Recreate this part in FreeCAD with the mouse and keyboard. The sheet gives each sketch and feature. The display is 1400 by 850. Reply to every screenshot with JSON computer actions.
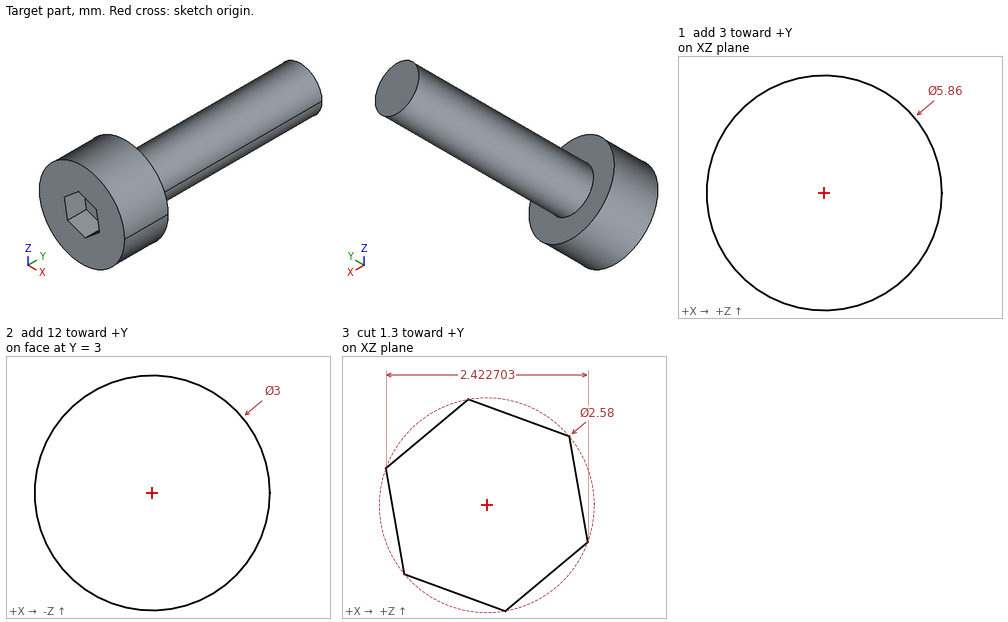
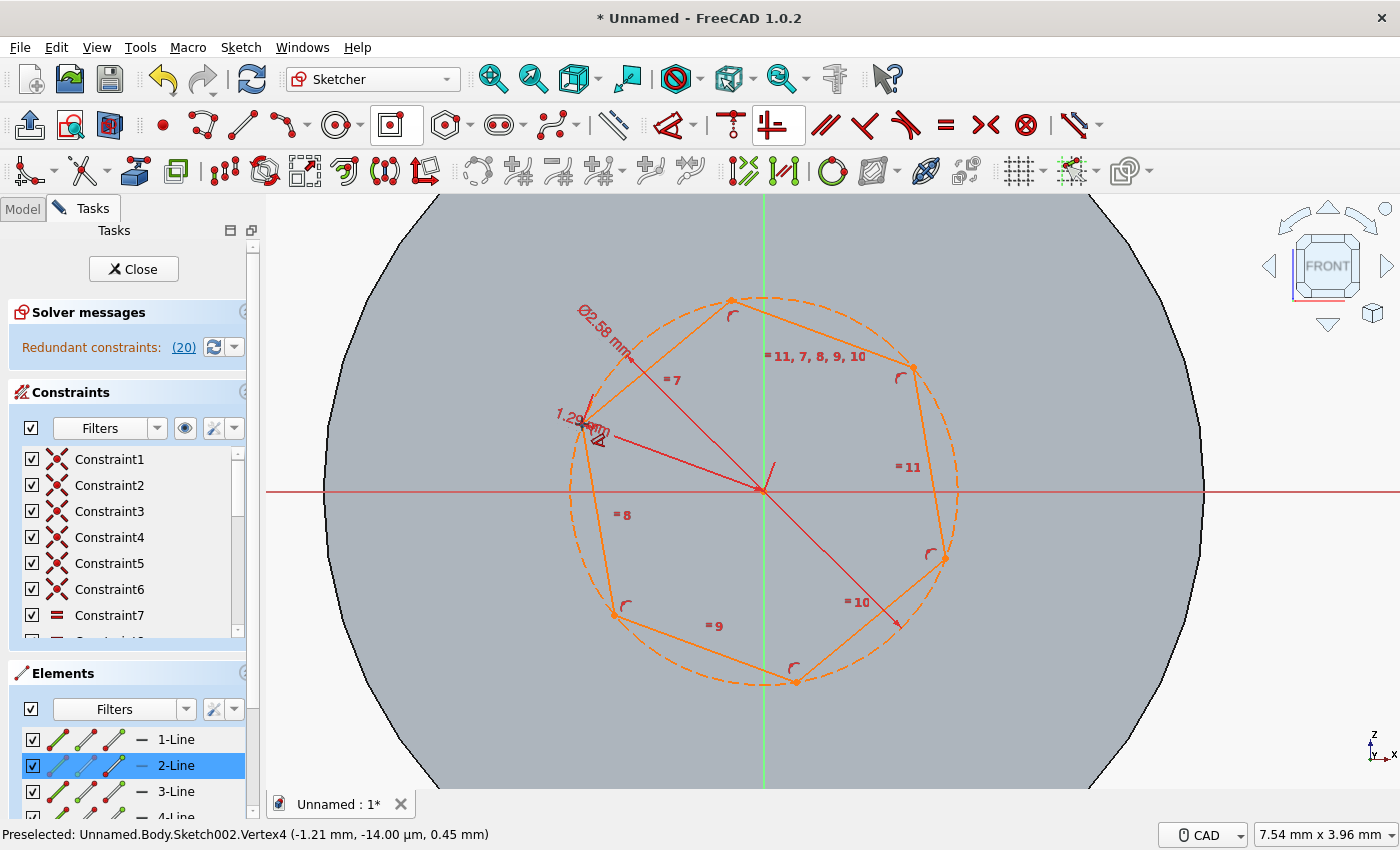
{"action": "left_click", "coordinate": [946, 559]}
{"action": "left_click", "coordinate": [680, 593]}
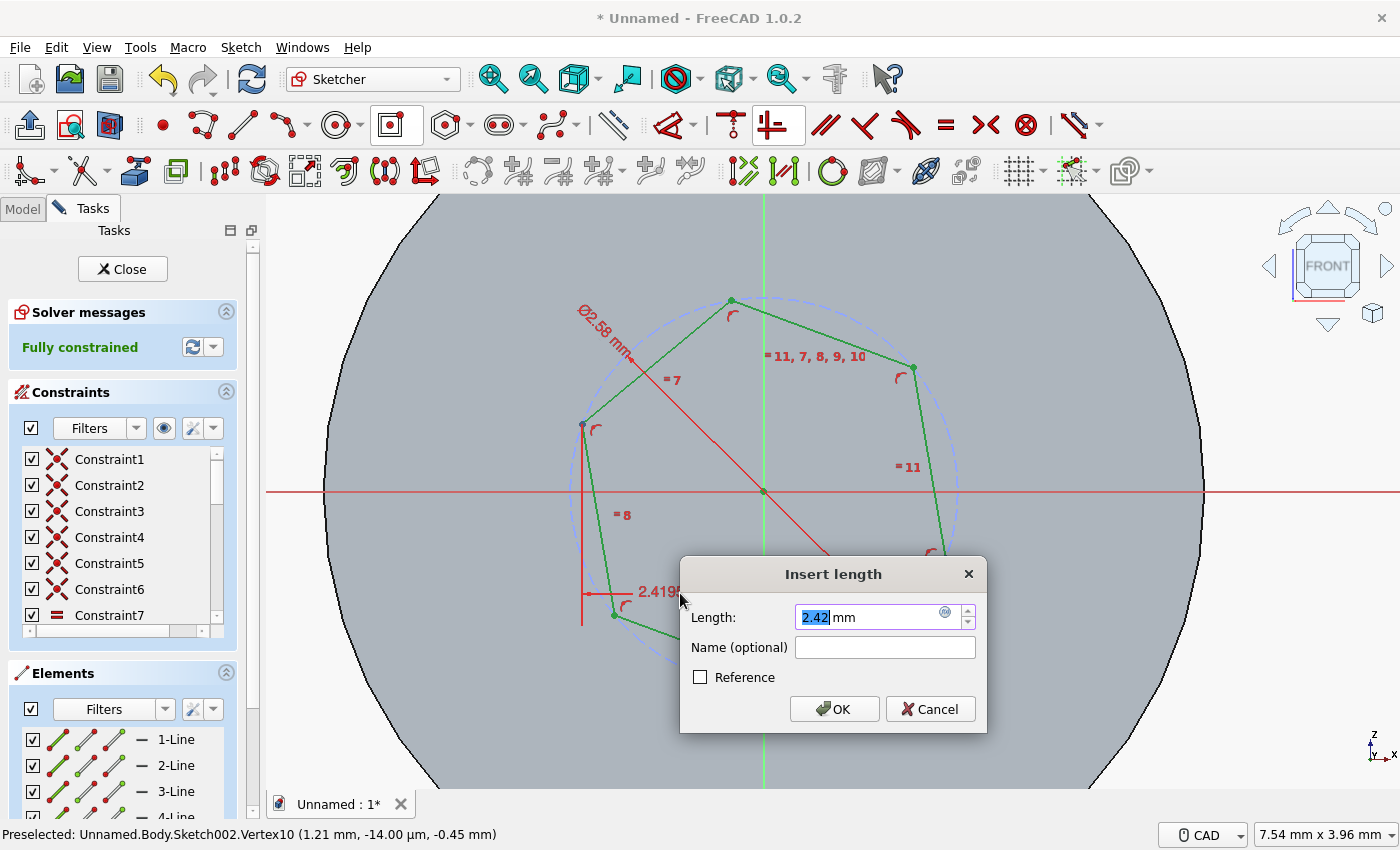
{"action": "type", "text": "2.422703"}
{"action": "key", "text": "Return"}
{"action": "key", "text": "Escape"}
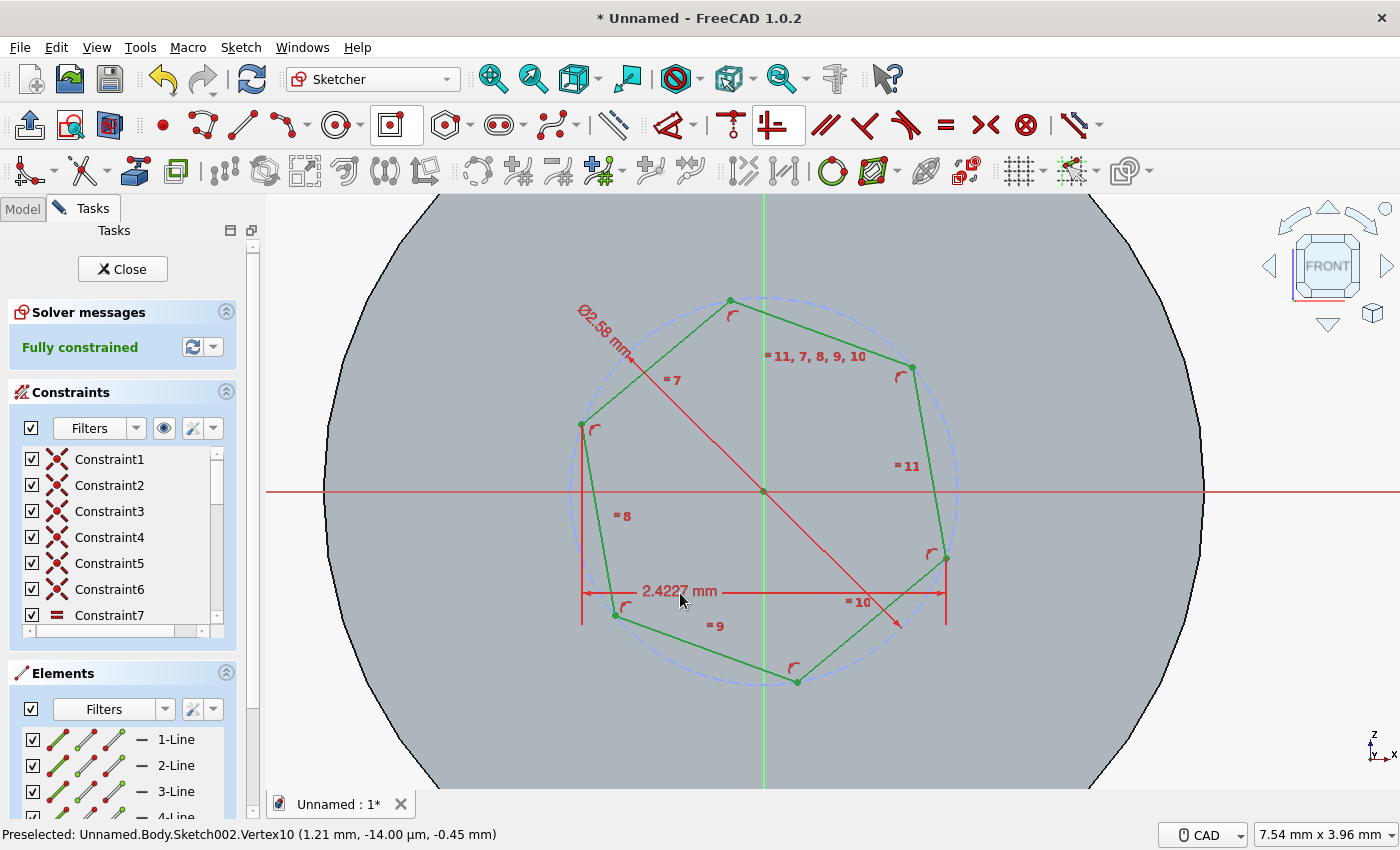
{"action": "left_click", "coordinate": [123, 269]}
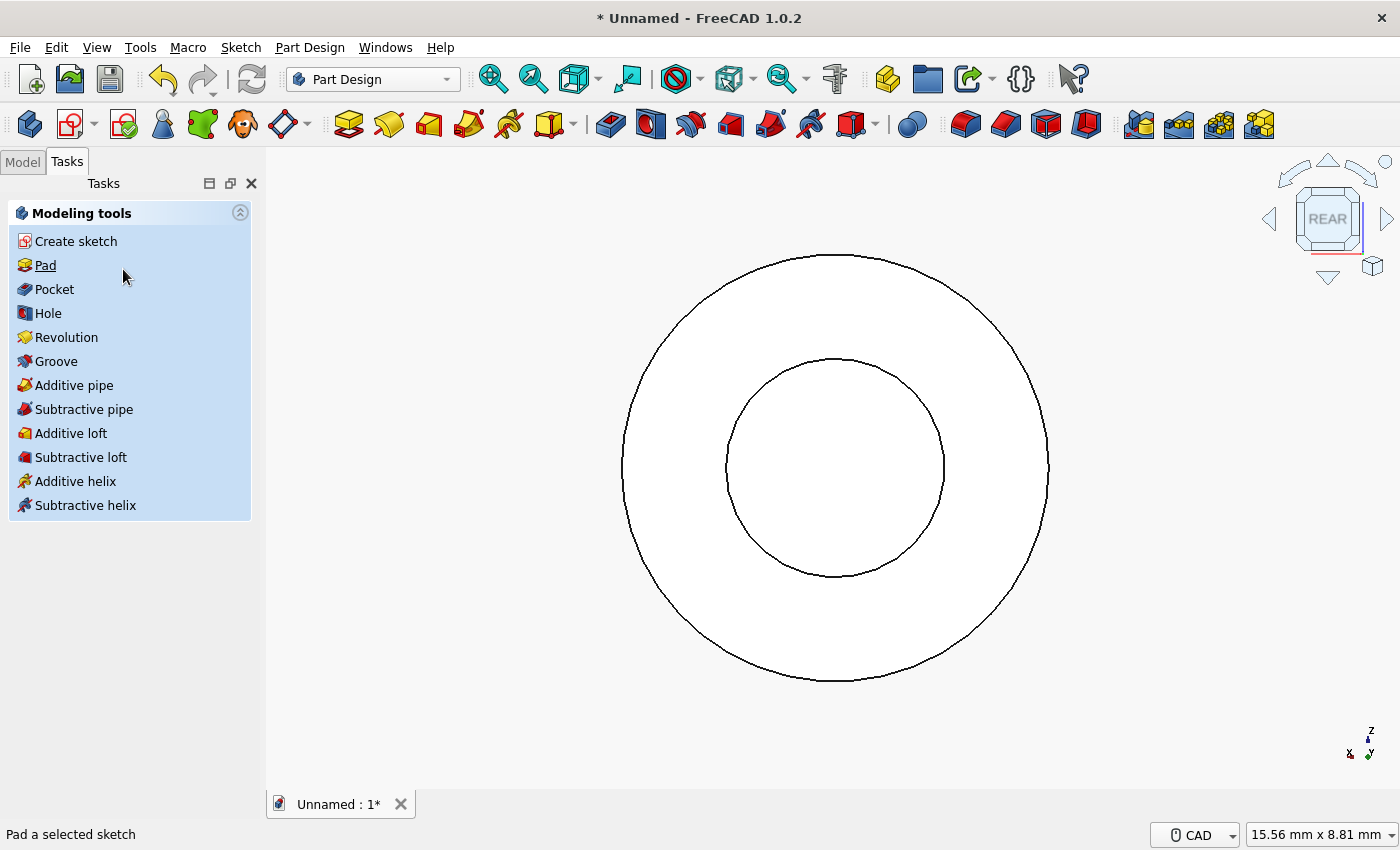
{"action": "left_click", "coordinate": [612, 124]}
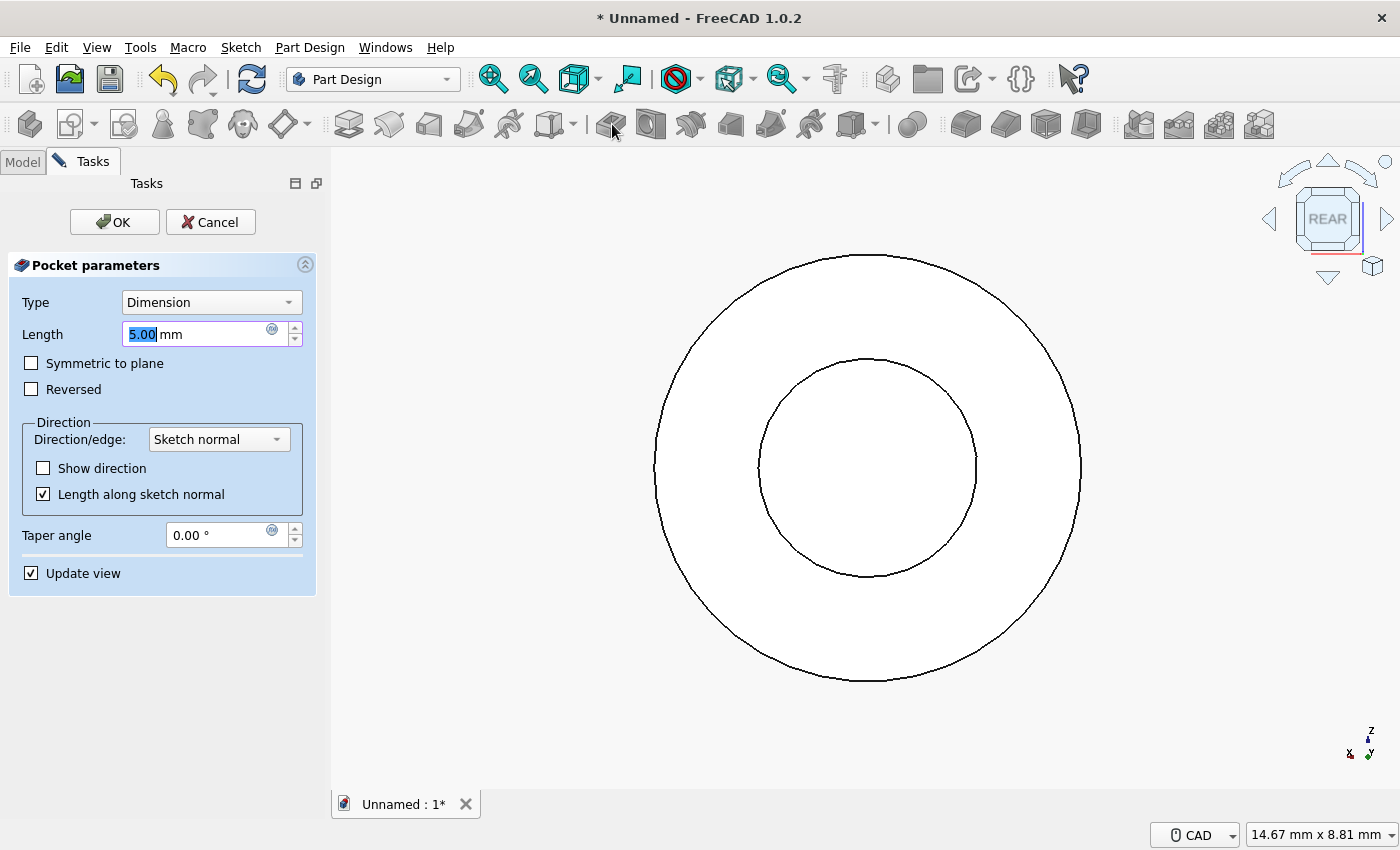
{"action": "type", "text": "1.3"}
{"action": "key", "text": "Tab"}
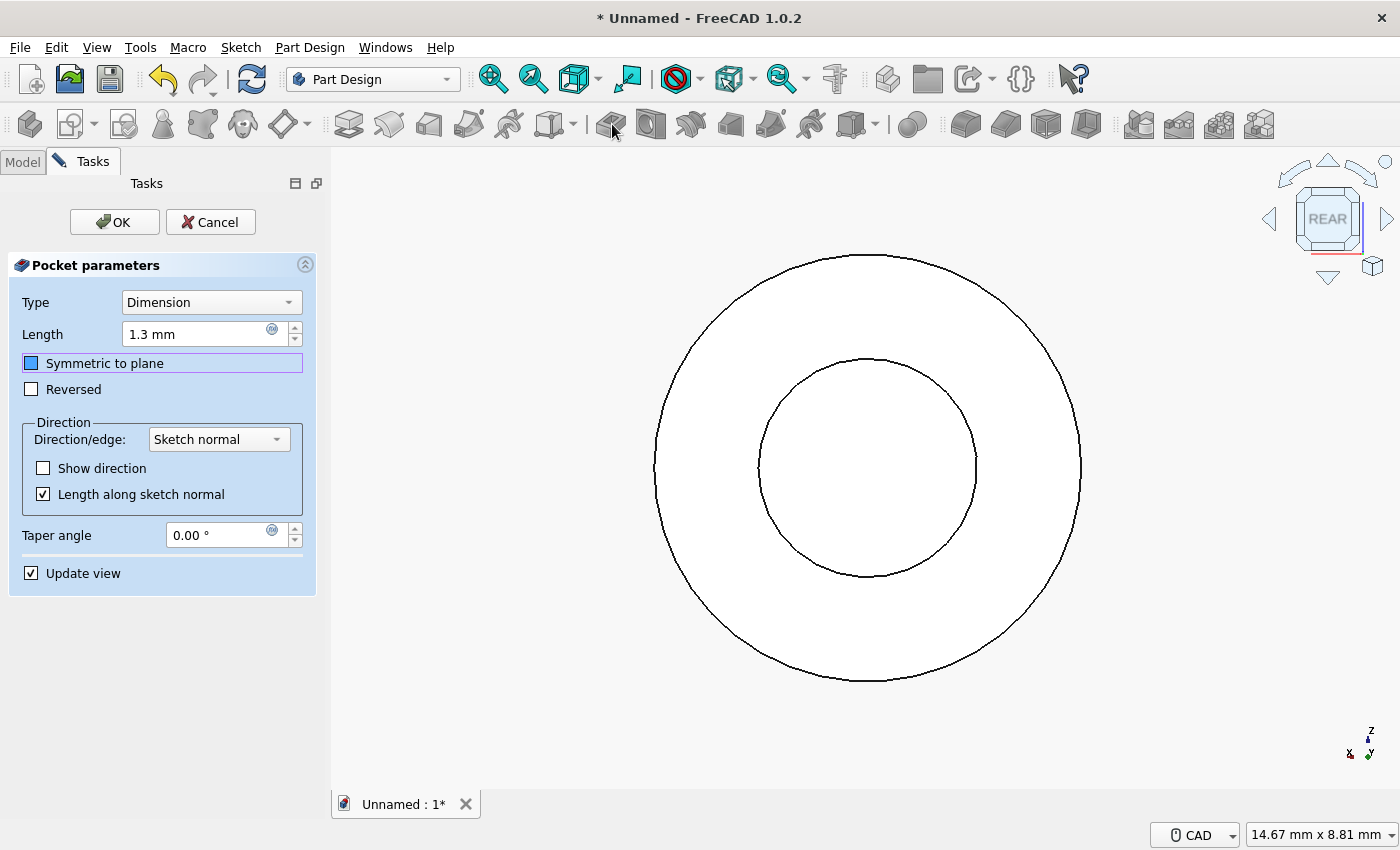
{"action": "left_click", "coordinate": [115, 222]}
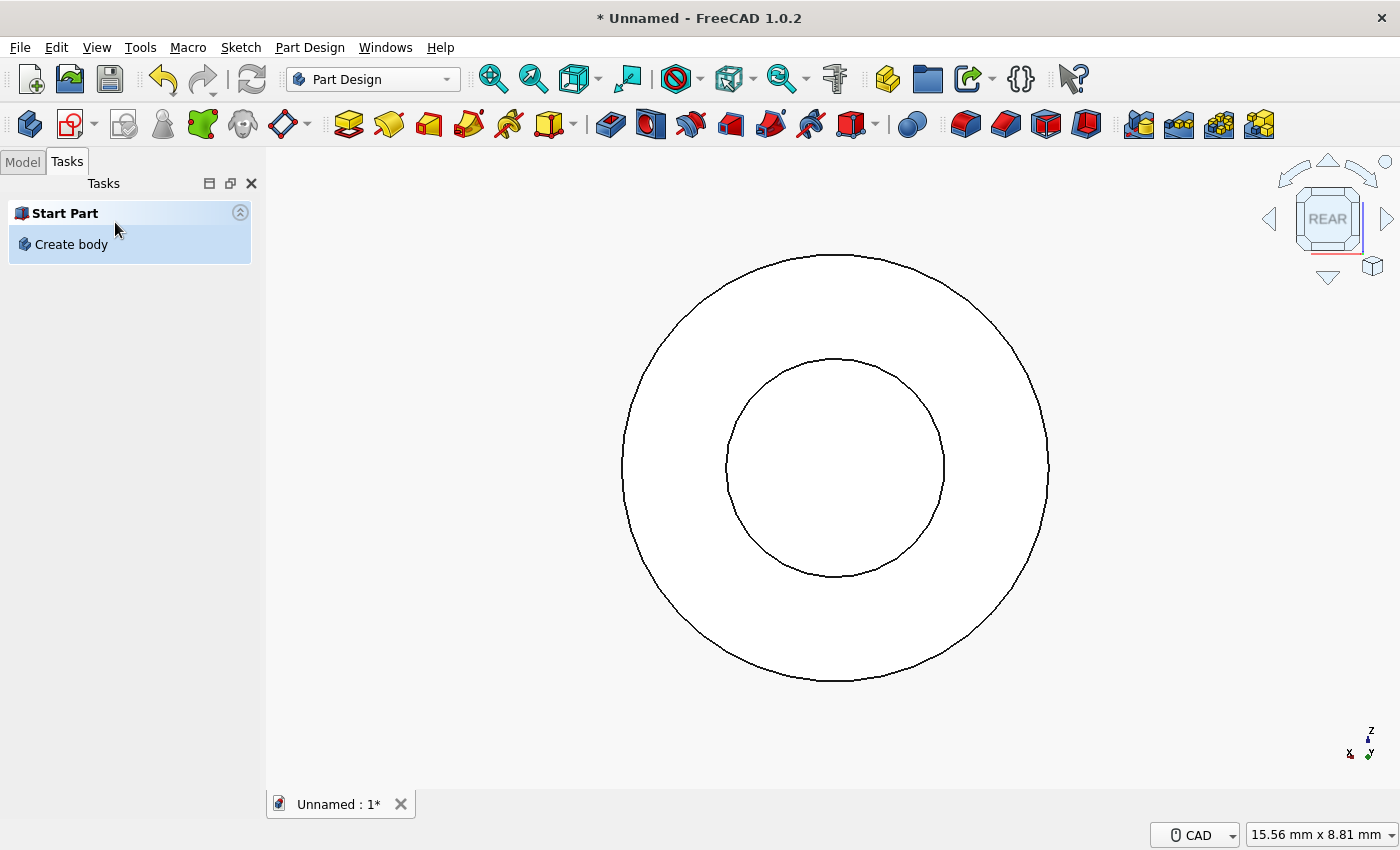
{"action": "key", "text": "0"}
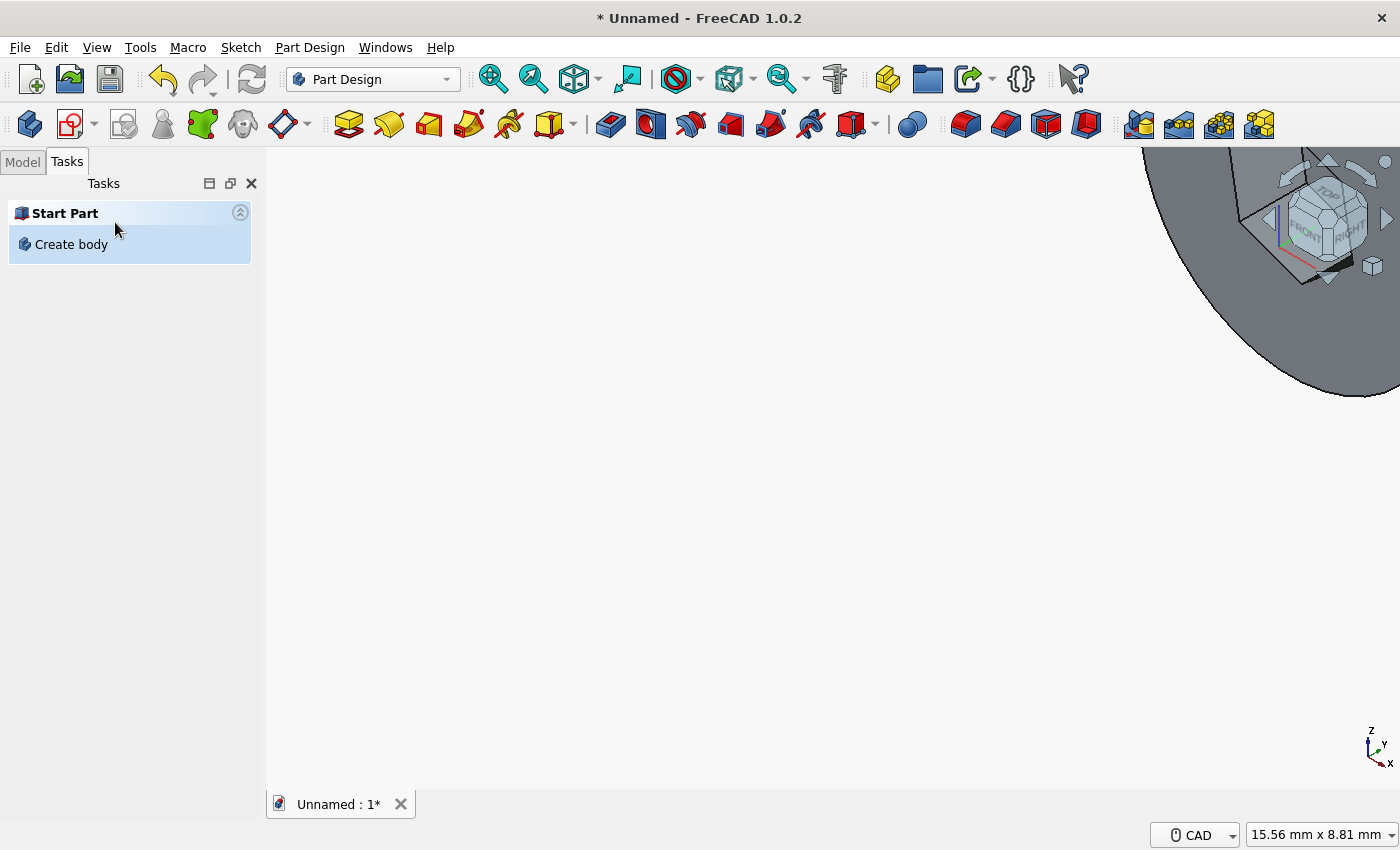
{"action": "left_click", "coordinate": [494, 80]}